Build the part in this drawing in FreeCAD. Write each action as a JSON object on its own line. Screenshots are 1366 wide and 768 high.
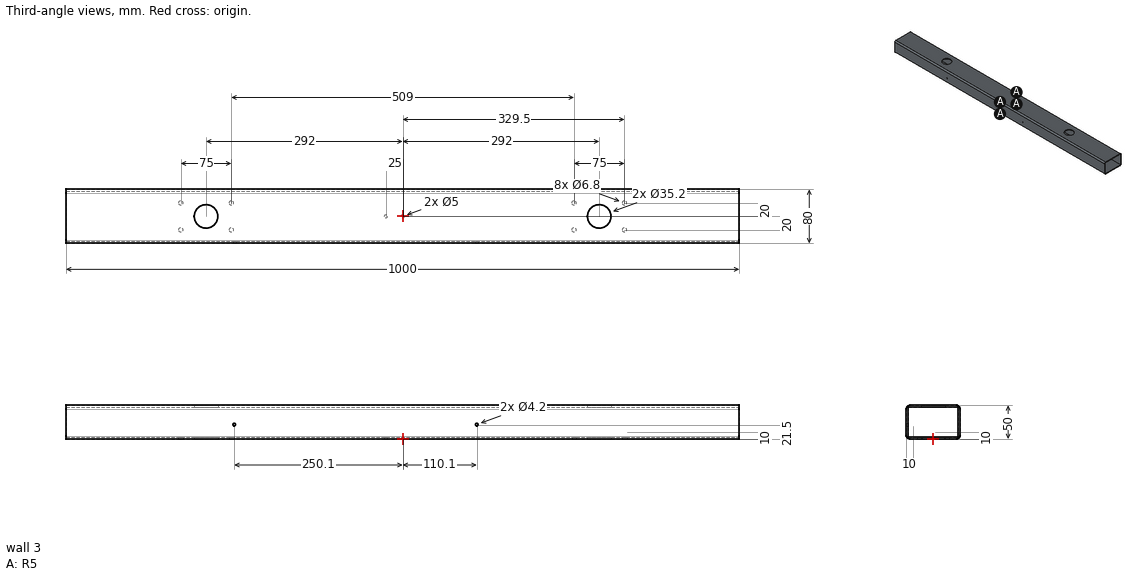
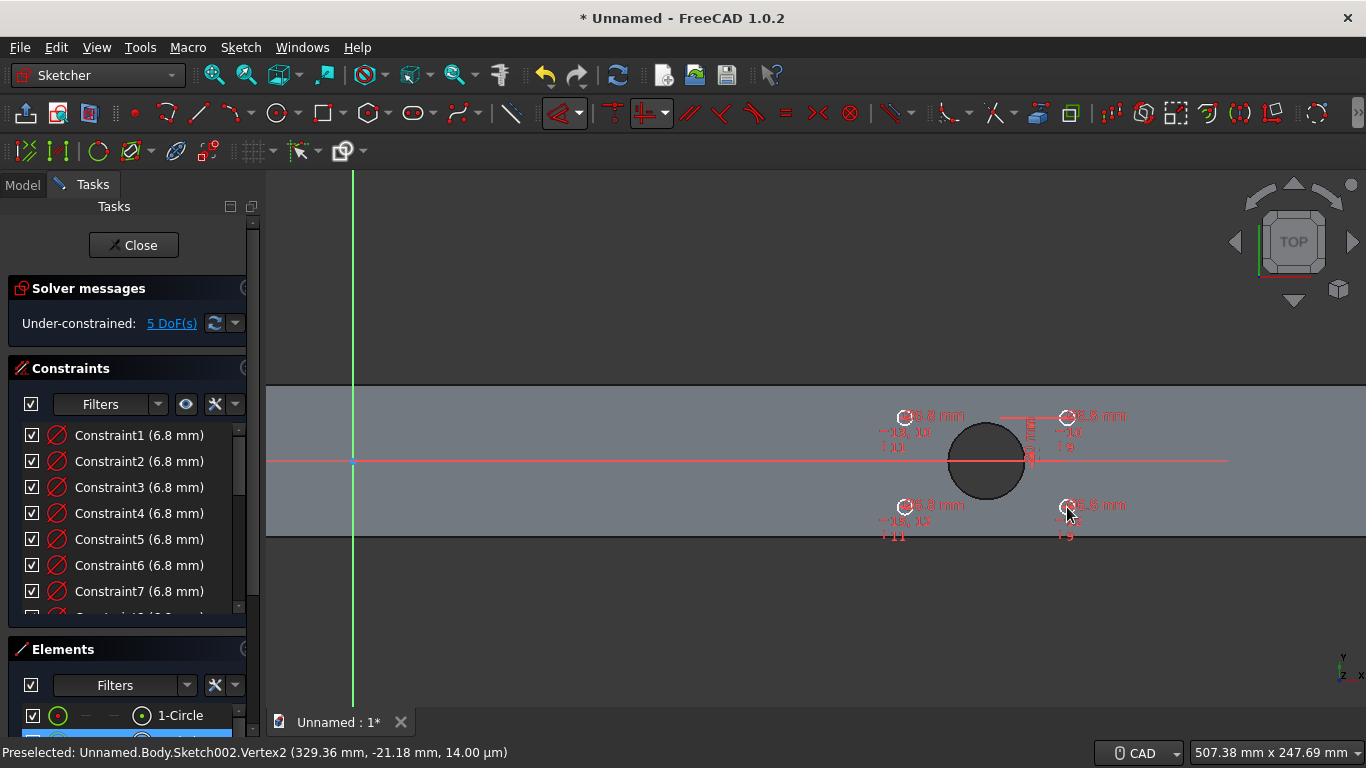
{"action": "key", "text": "i"}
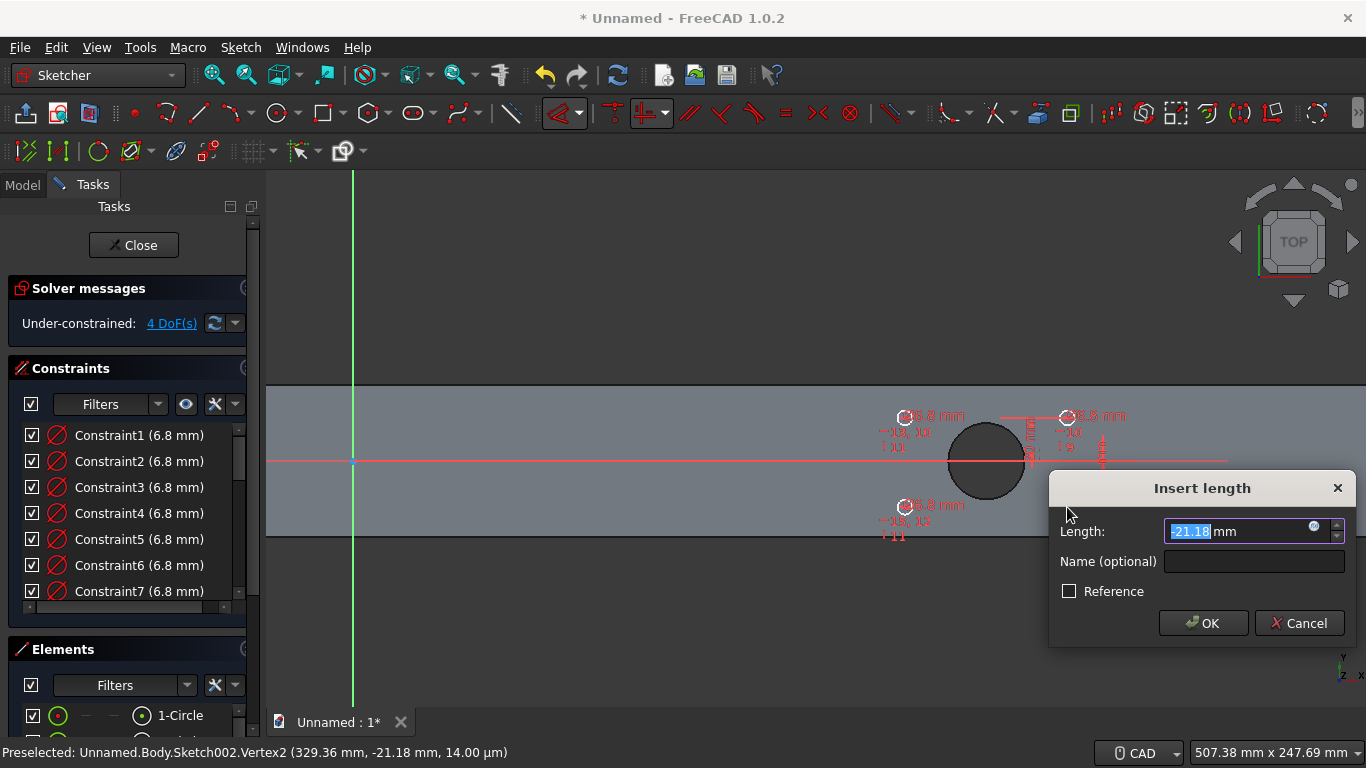
{"action": "type", "text": "-20"}
{"action": "key", "text": "Return"}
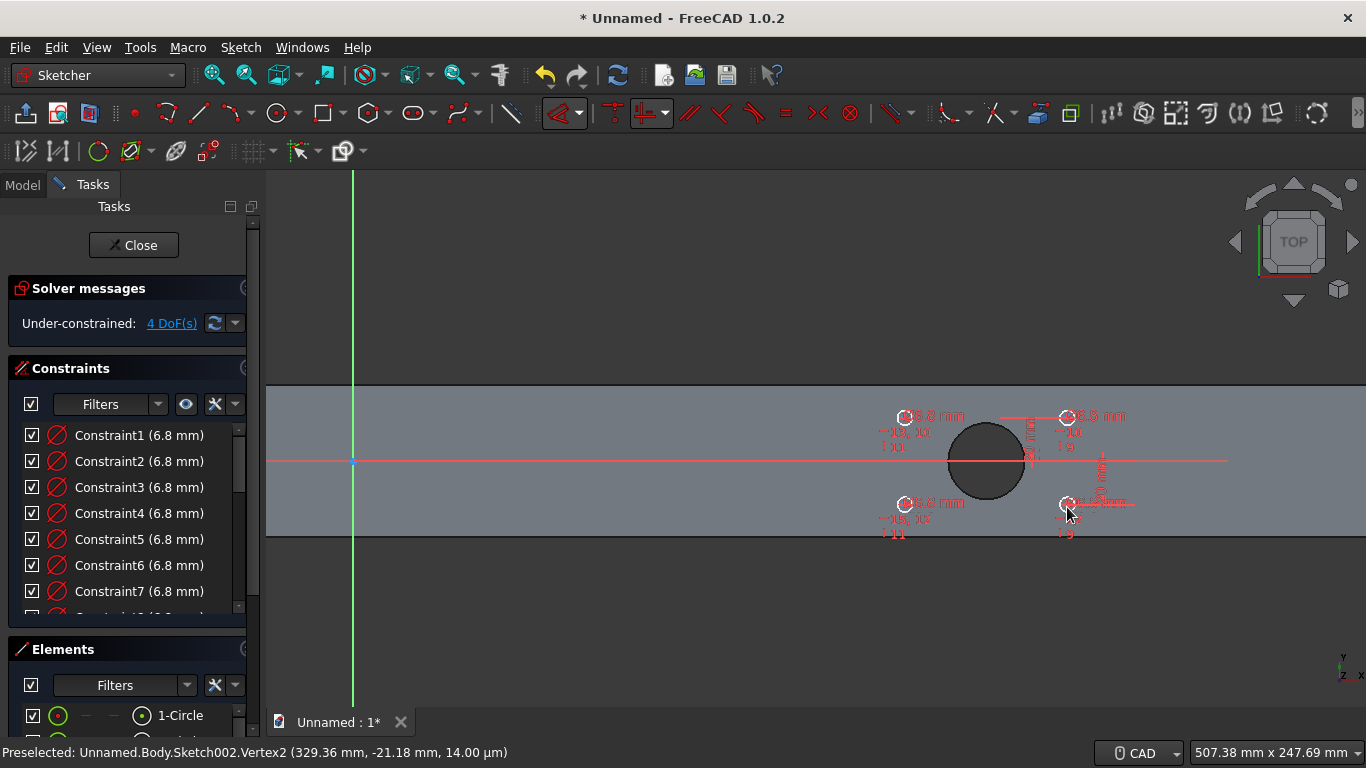
{"action": "left_click", "coordinate": [1067, 418]}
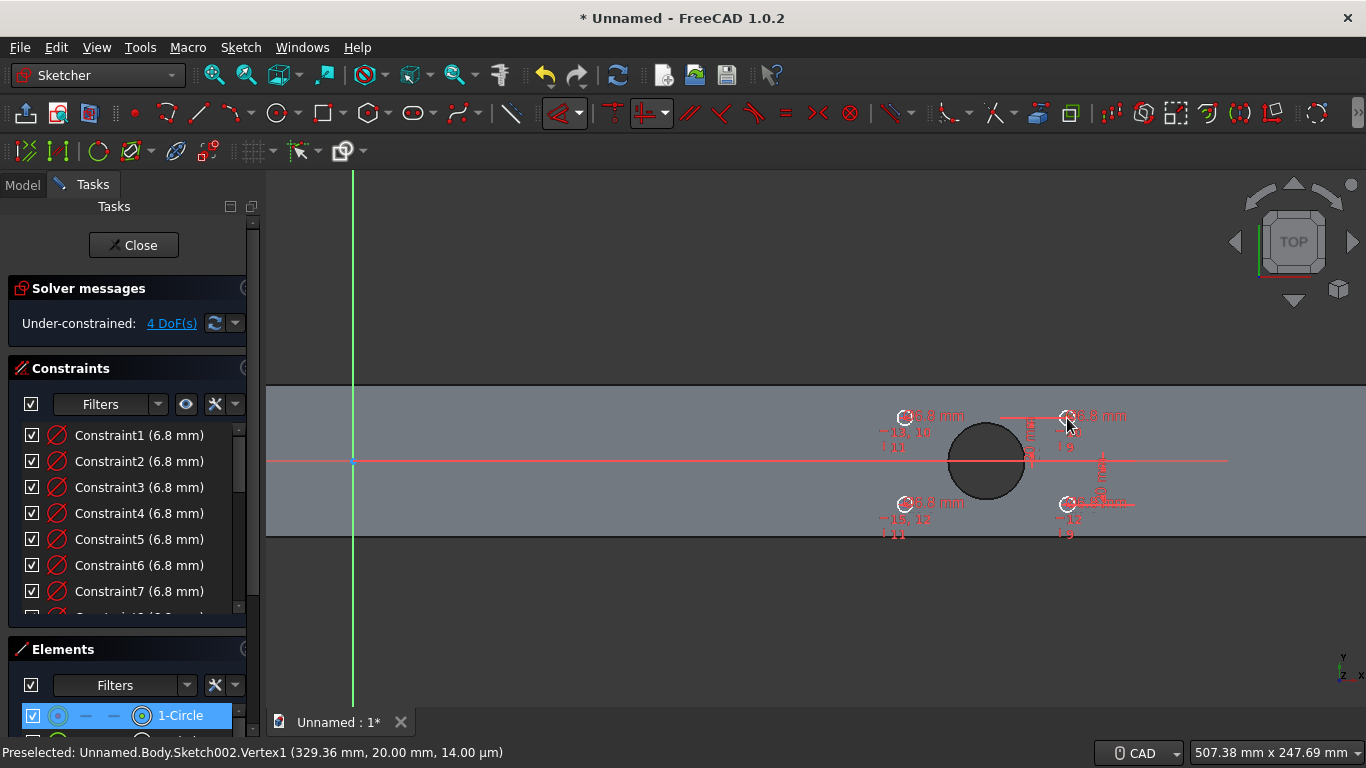
{"action": "left_click", "coordinate": [905, 418]}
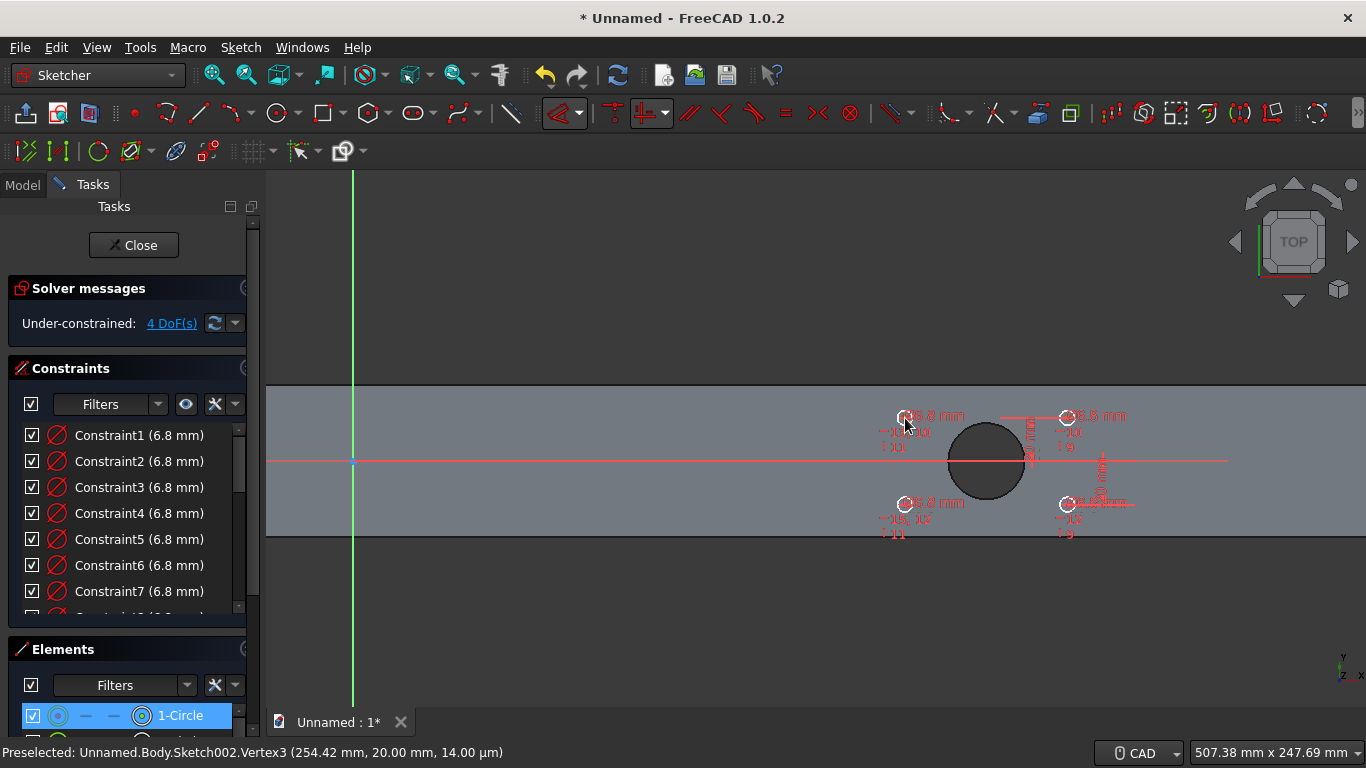
{"action": "left_click", "coordinate": [582, 114]}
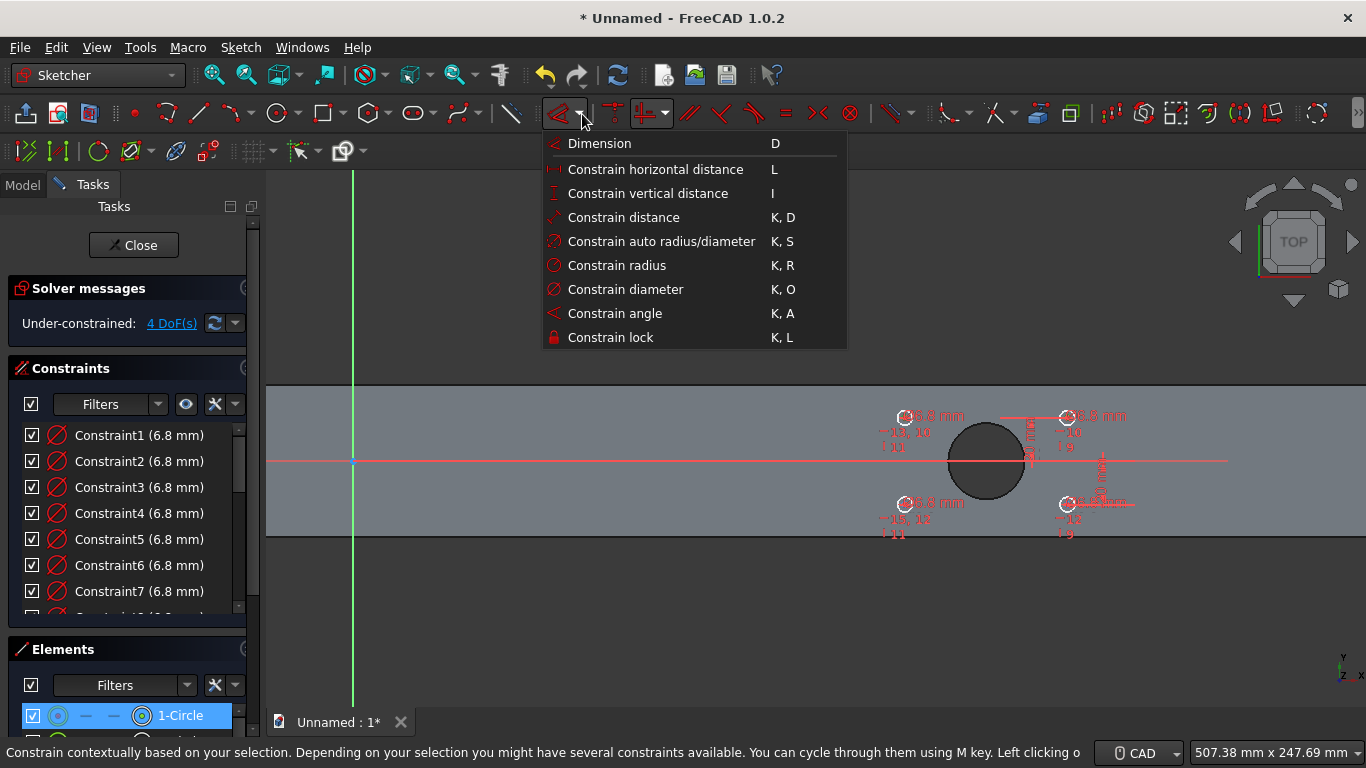
{"action": "left_click", "coordinate": [695, 169]}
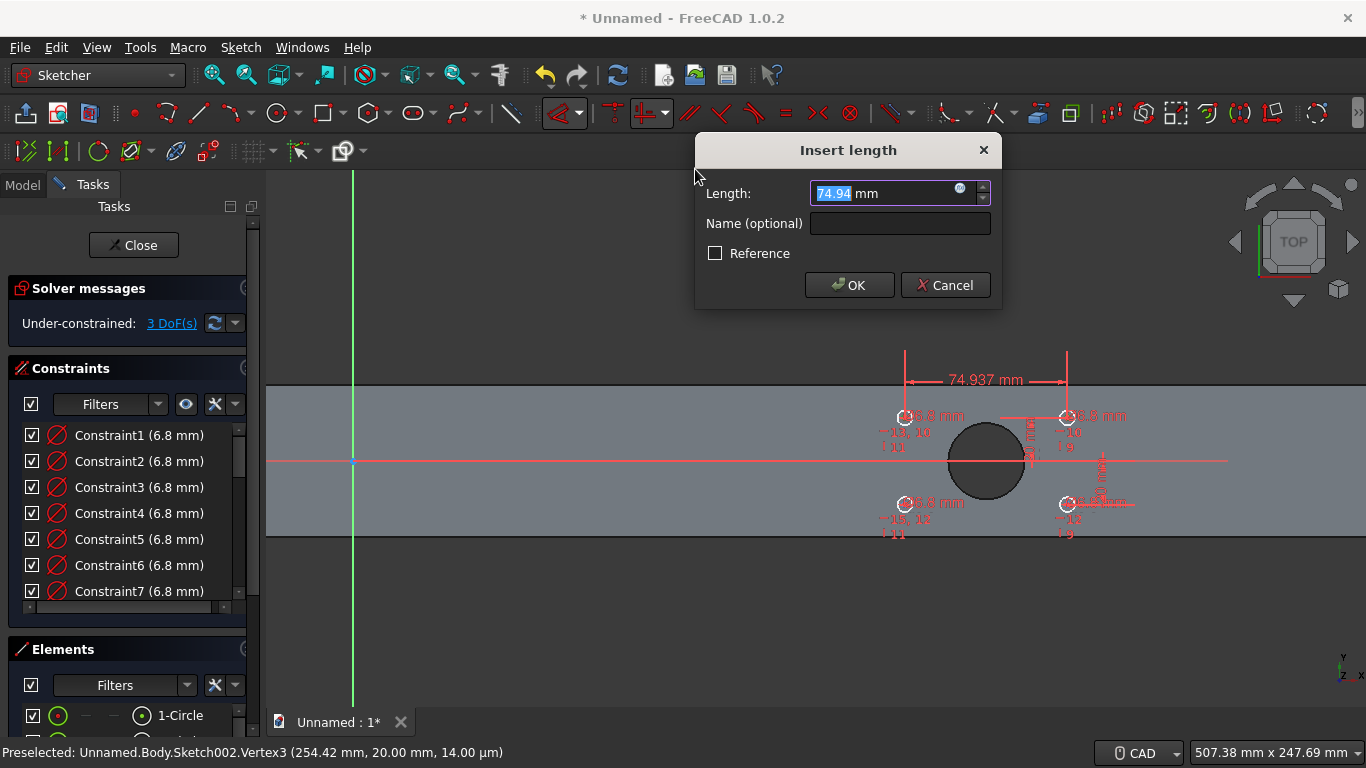
{"action": "type", "text": "75"}
{"action": "key", "text": "Return"}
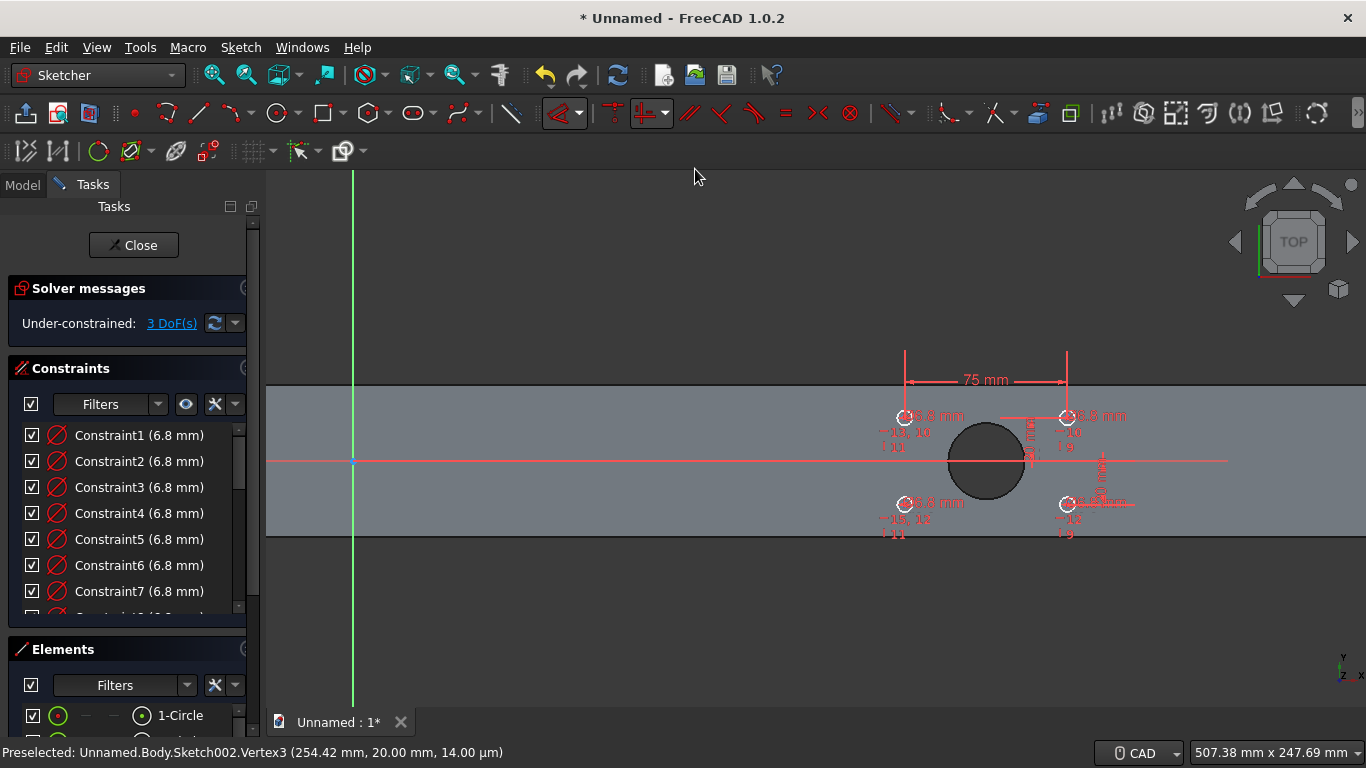
{"action": "scroll", "coordinate": [1069, 420], "scroll_direction": "down", "scroll_amount": 4}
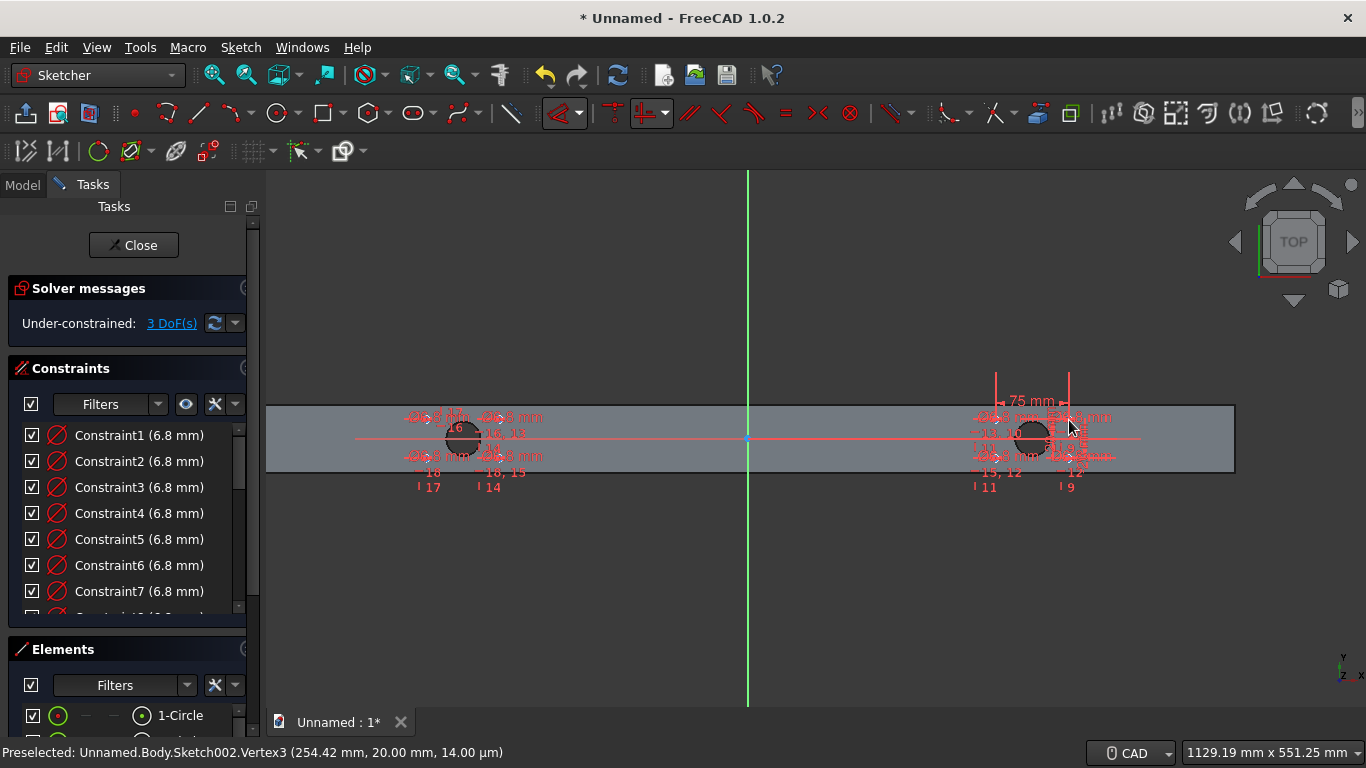
{"action": "left_click", "coordinate": [500, 419]}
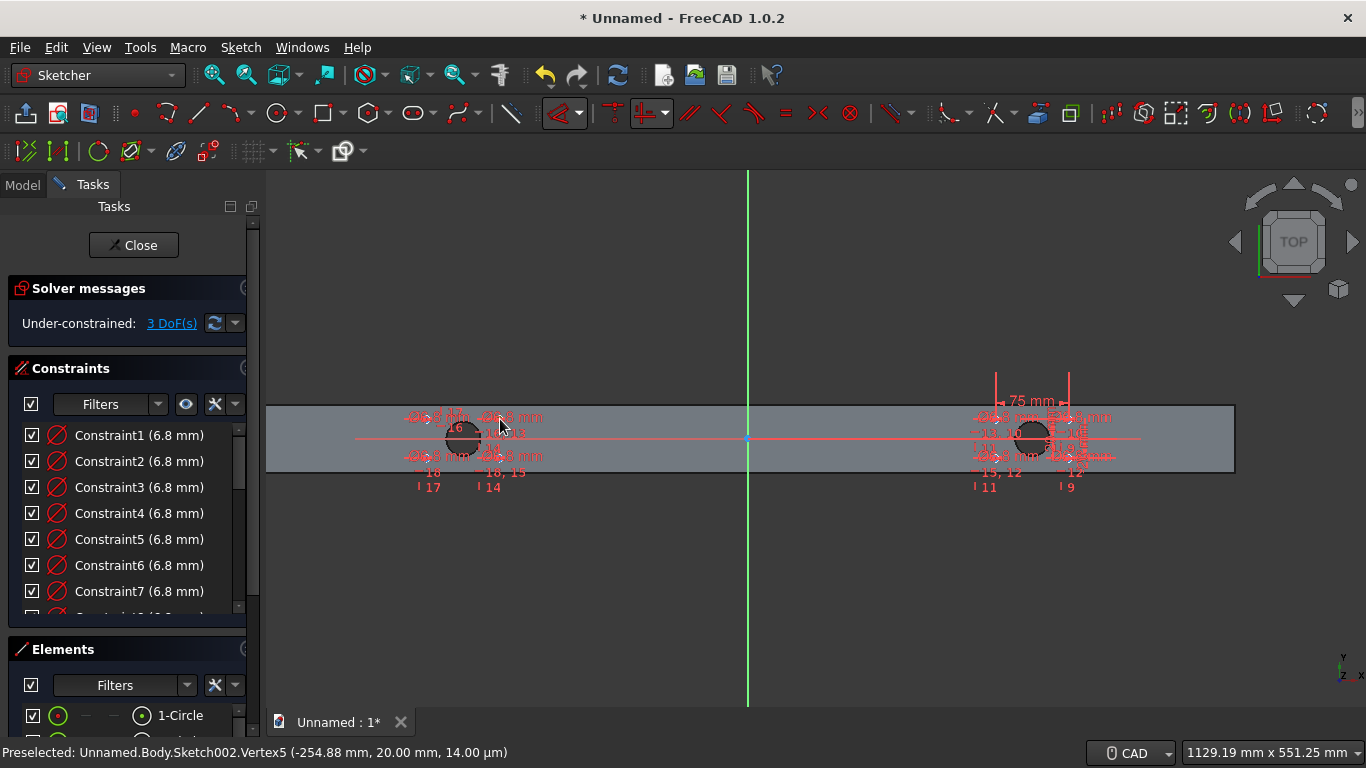
{"action": "left_click", "coordinate": [427, 419]}